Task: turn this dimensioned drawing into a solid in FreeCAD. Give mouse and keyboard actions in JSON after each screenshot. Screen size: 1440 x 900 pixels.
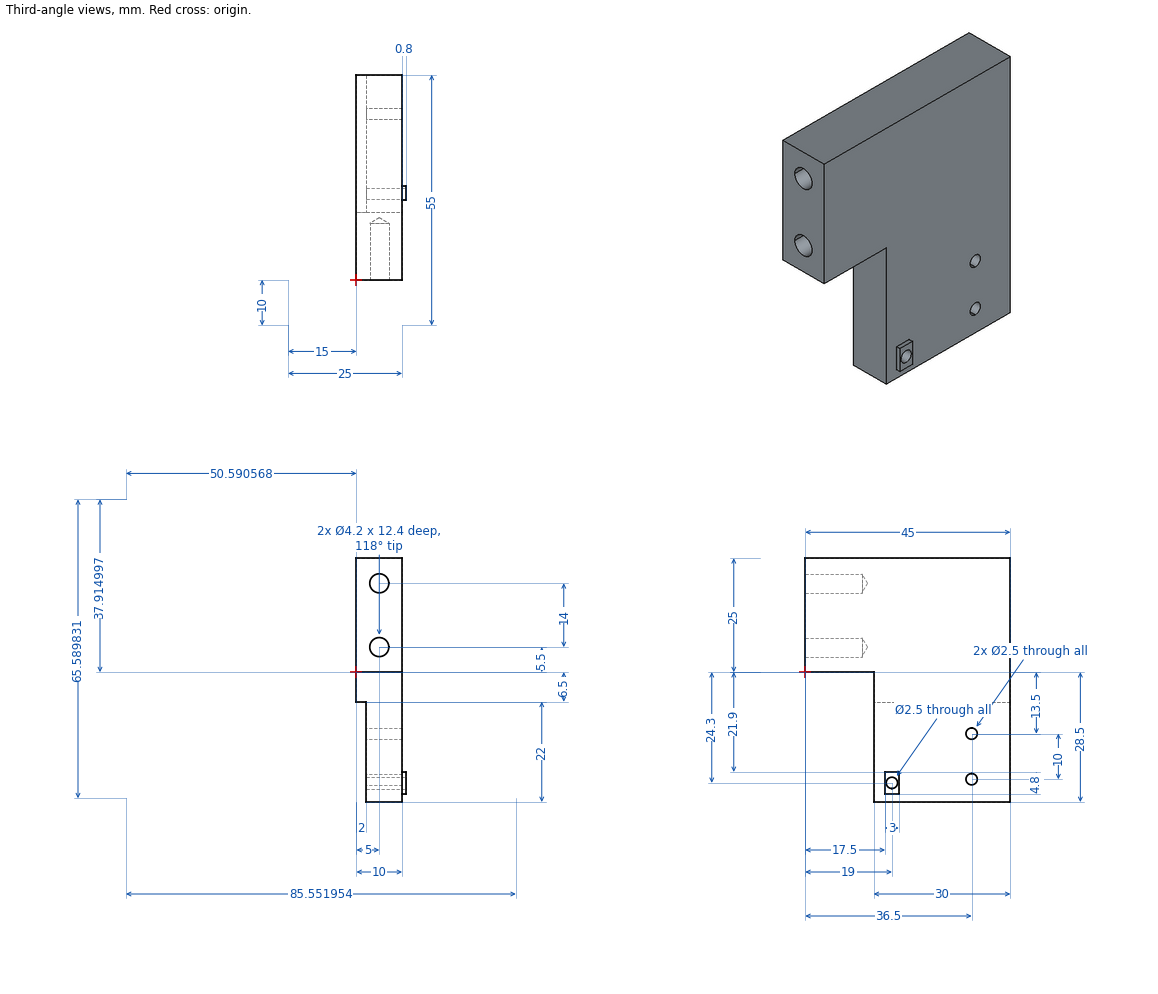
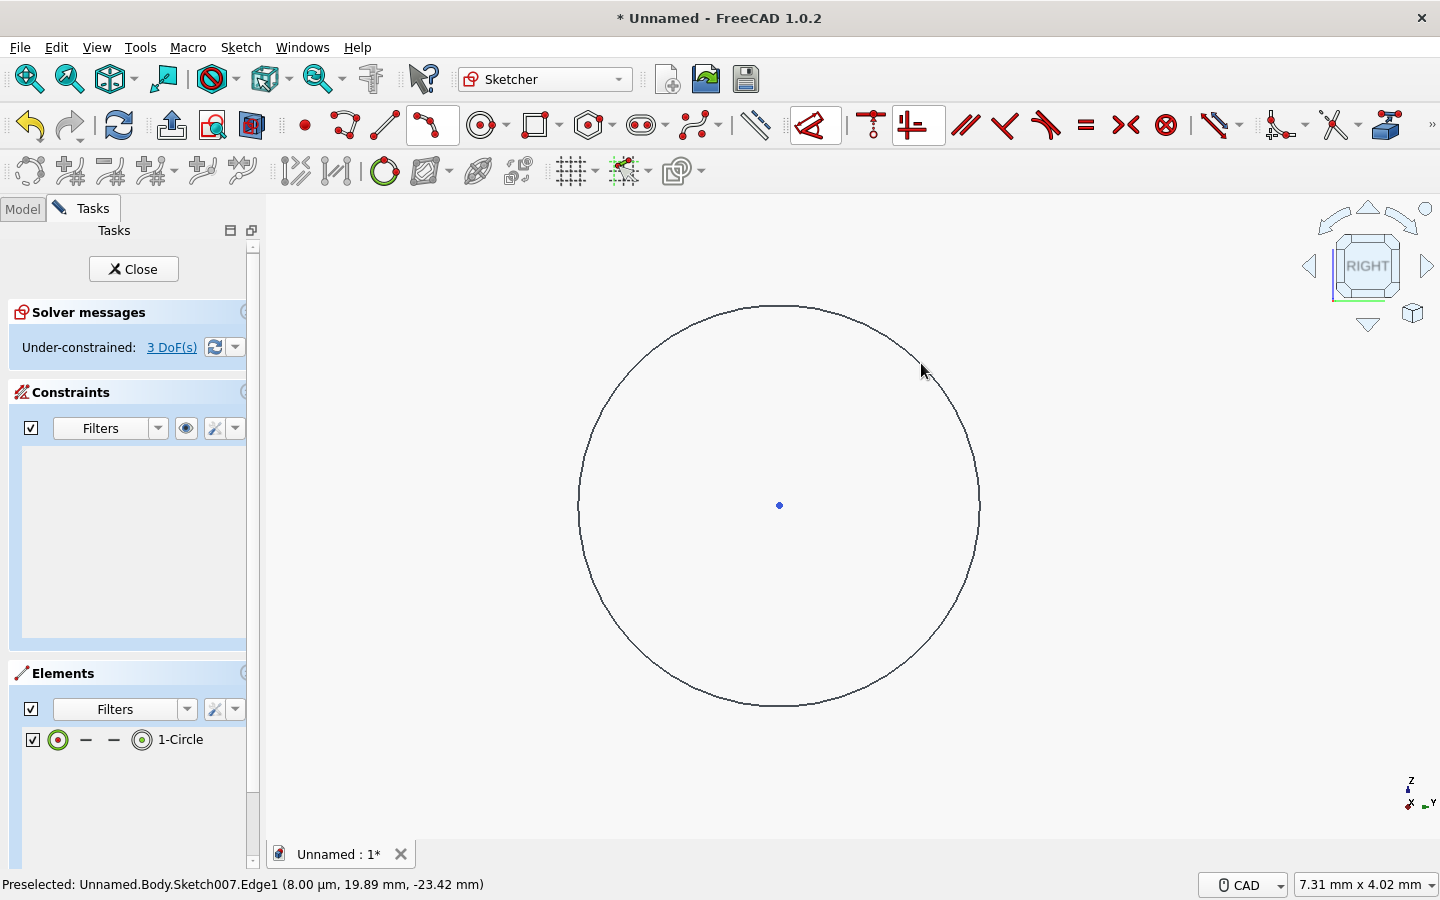
{"action": "left_click", "coordinate": [921, 364]}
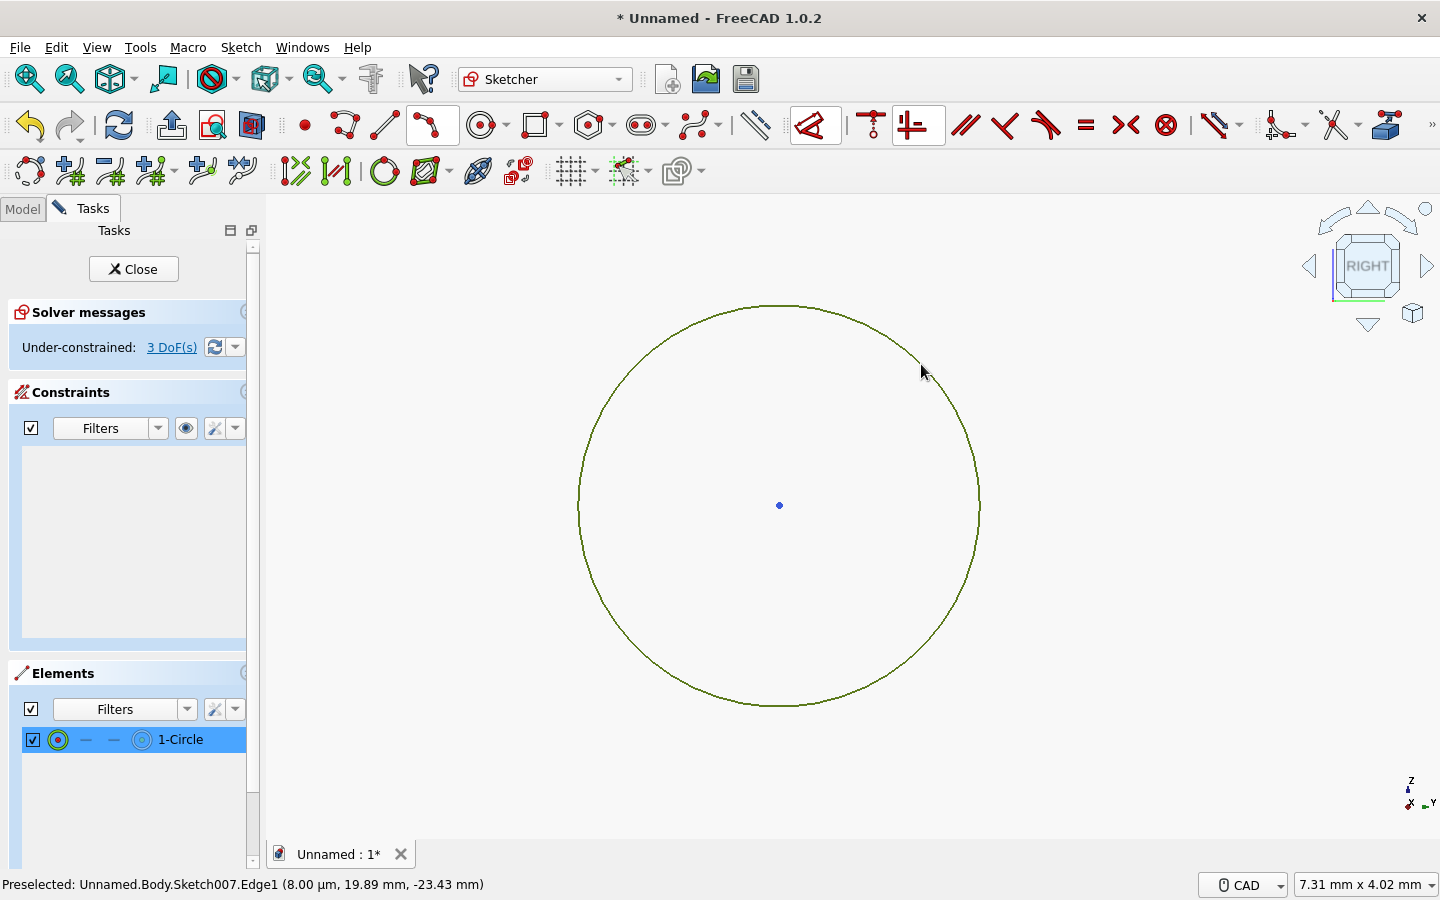
{"action": "left_click", "coordinate": [836, 126]}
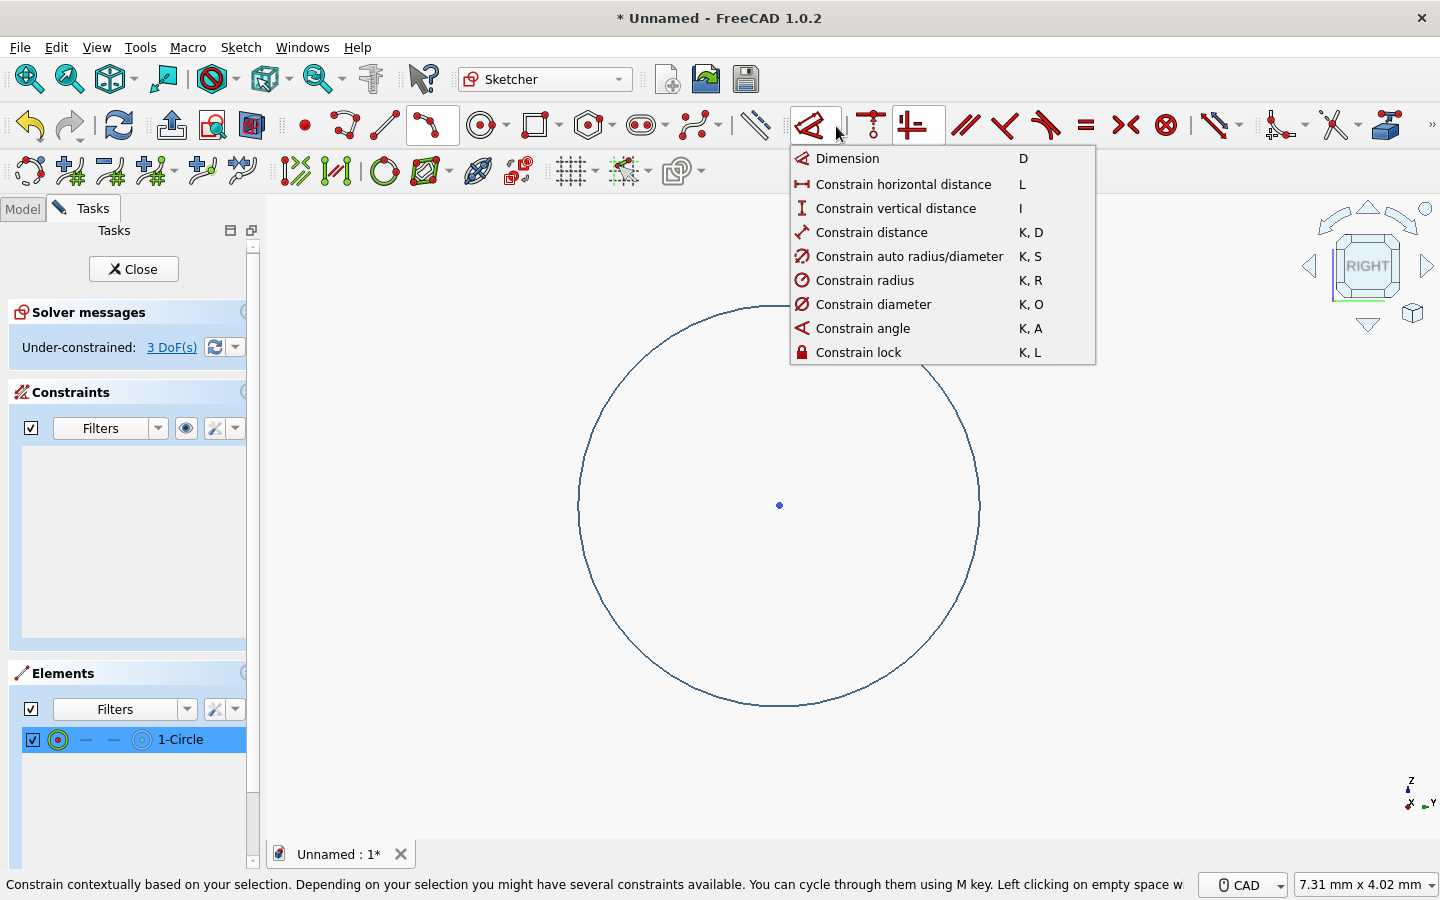
{"action": "left_click", "coordinate": [943, 304]}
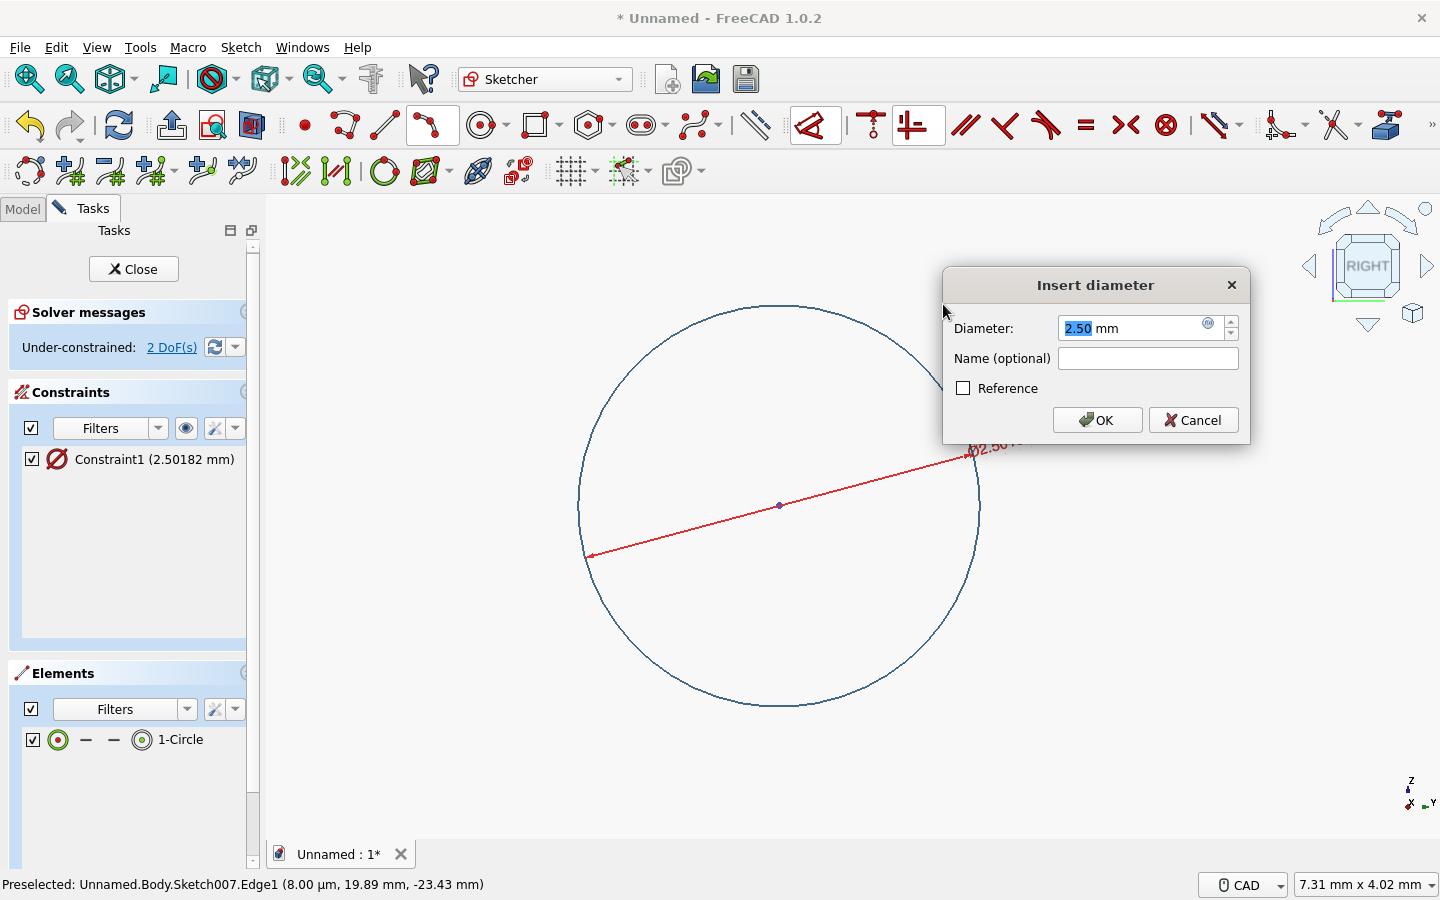
{"action": "type", "text": "2.5"}
{"action": "key", "text": "Return"}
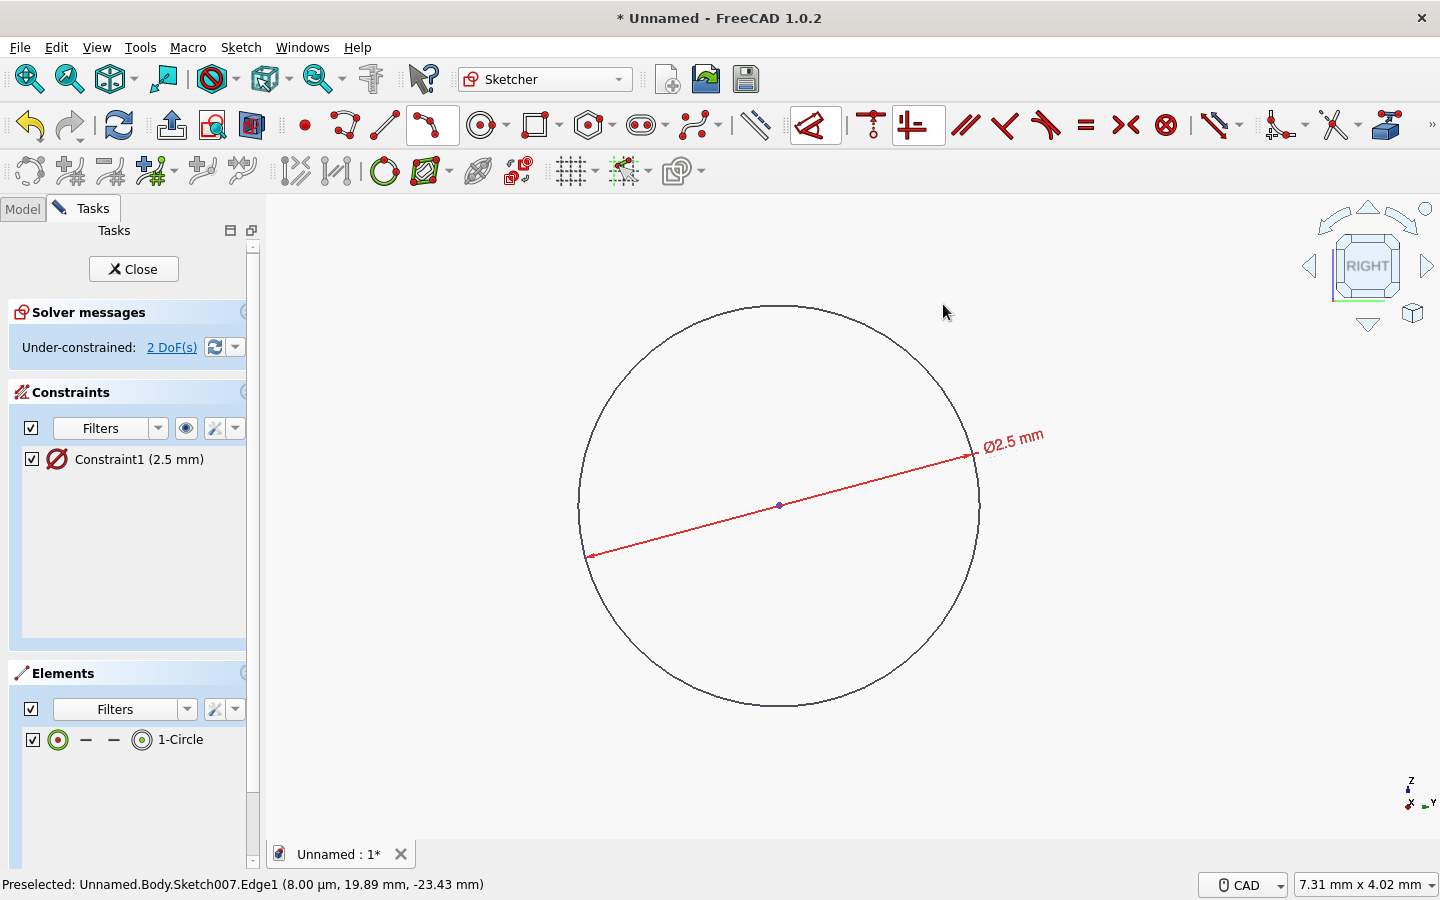
{"action": "left_click", "coordinate": [779, 506]}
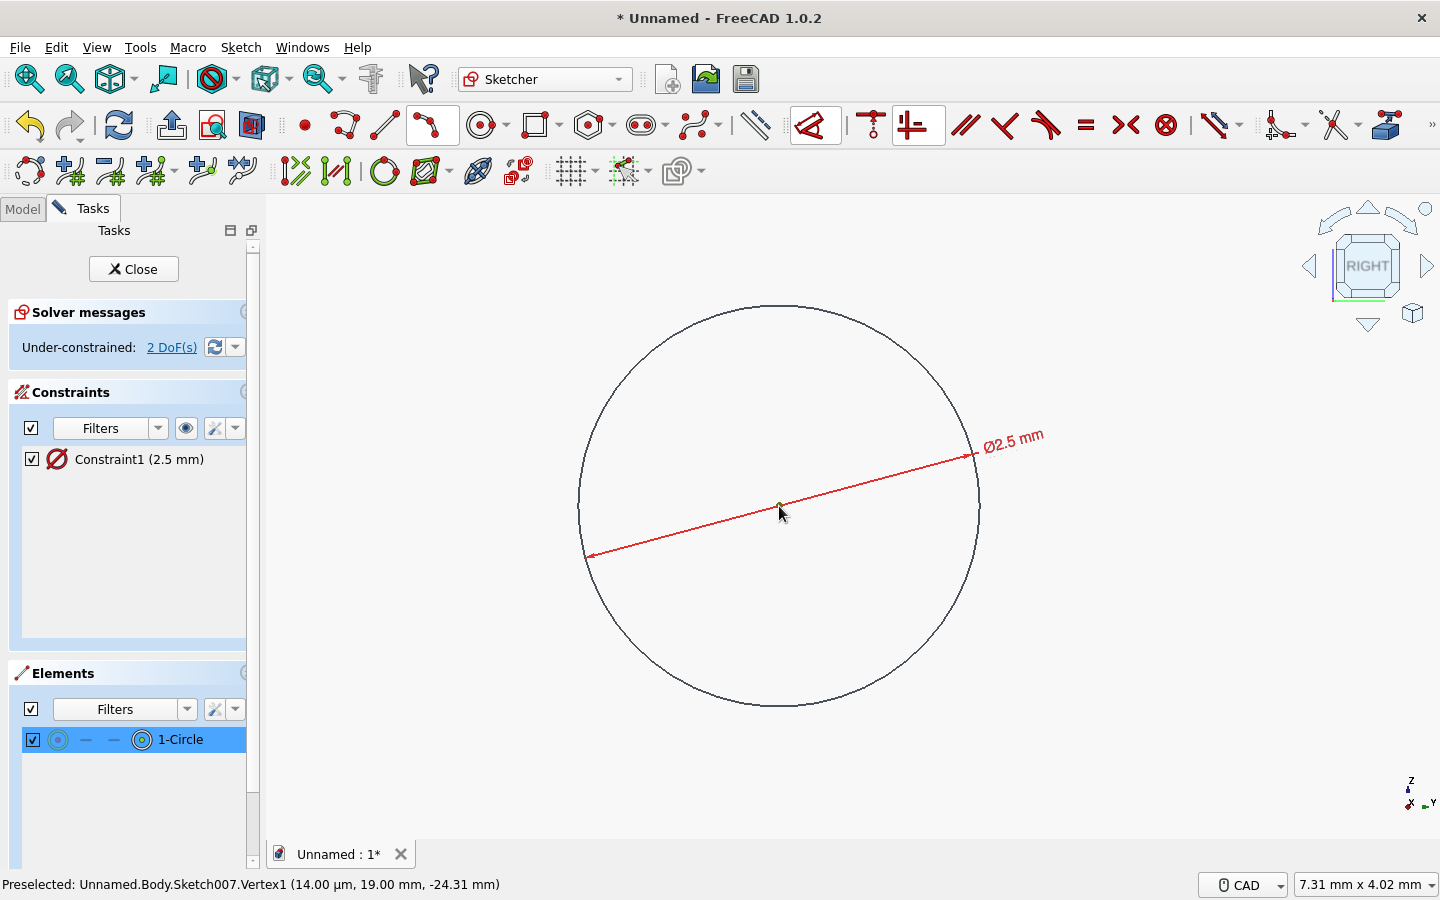
{"action": "key", "text": "l"}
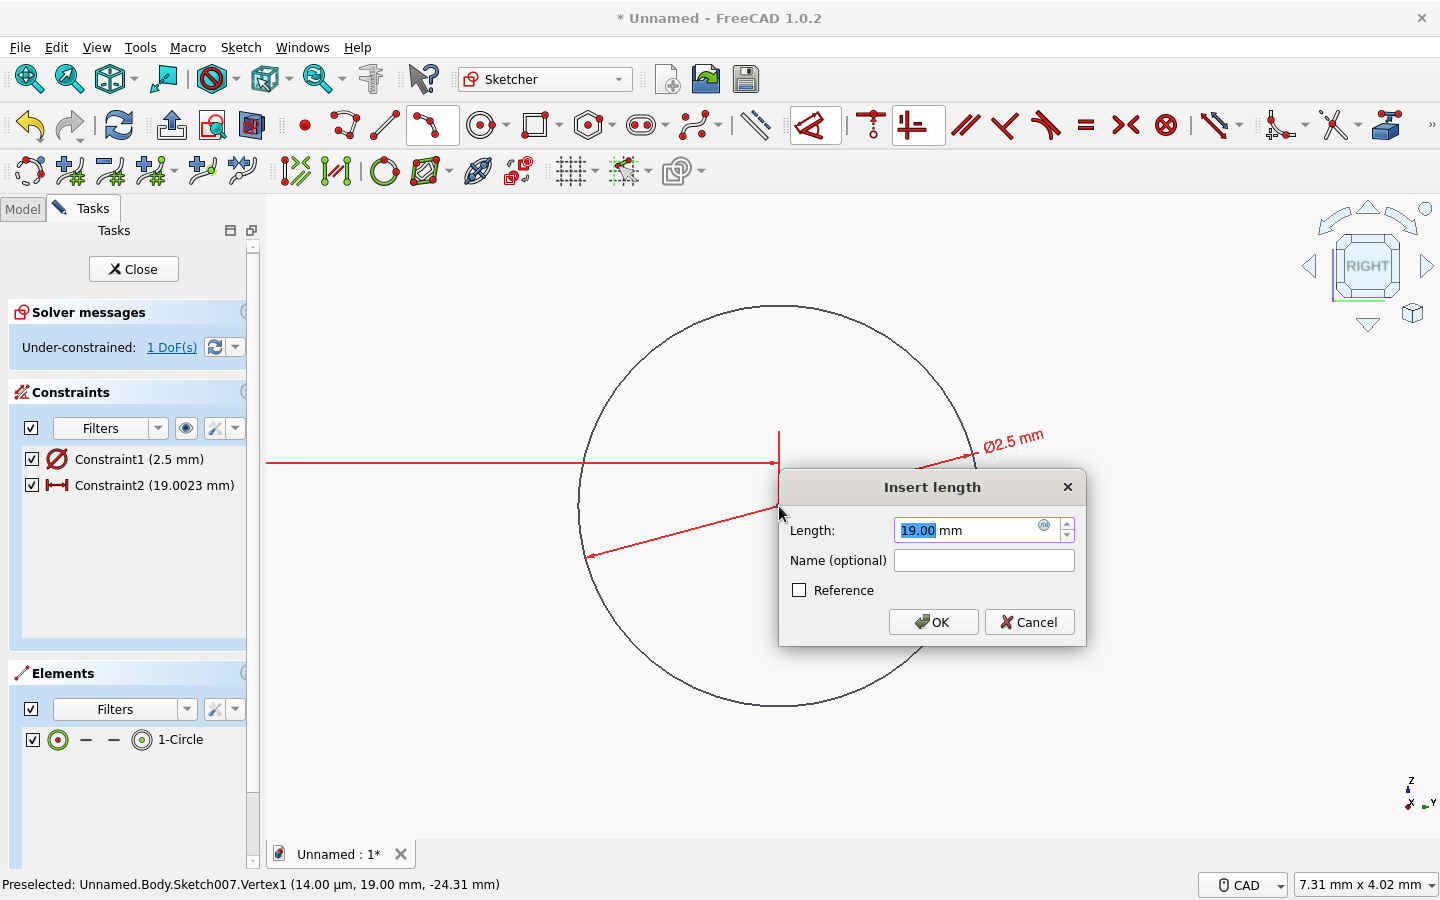
{"action": "type", "text": "19"}
{"action": "key", "text": "Return"}